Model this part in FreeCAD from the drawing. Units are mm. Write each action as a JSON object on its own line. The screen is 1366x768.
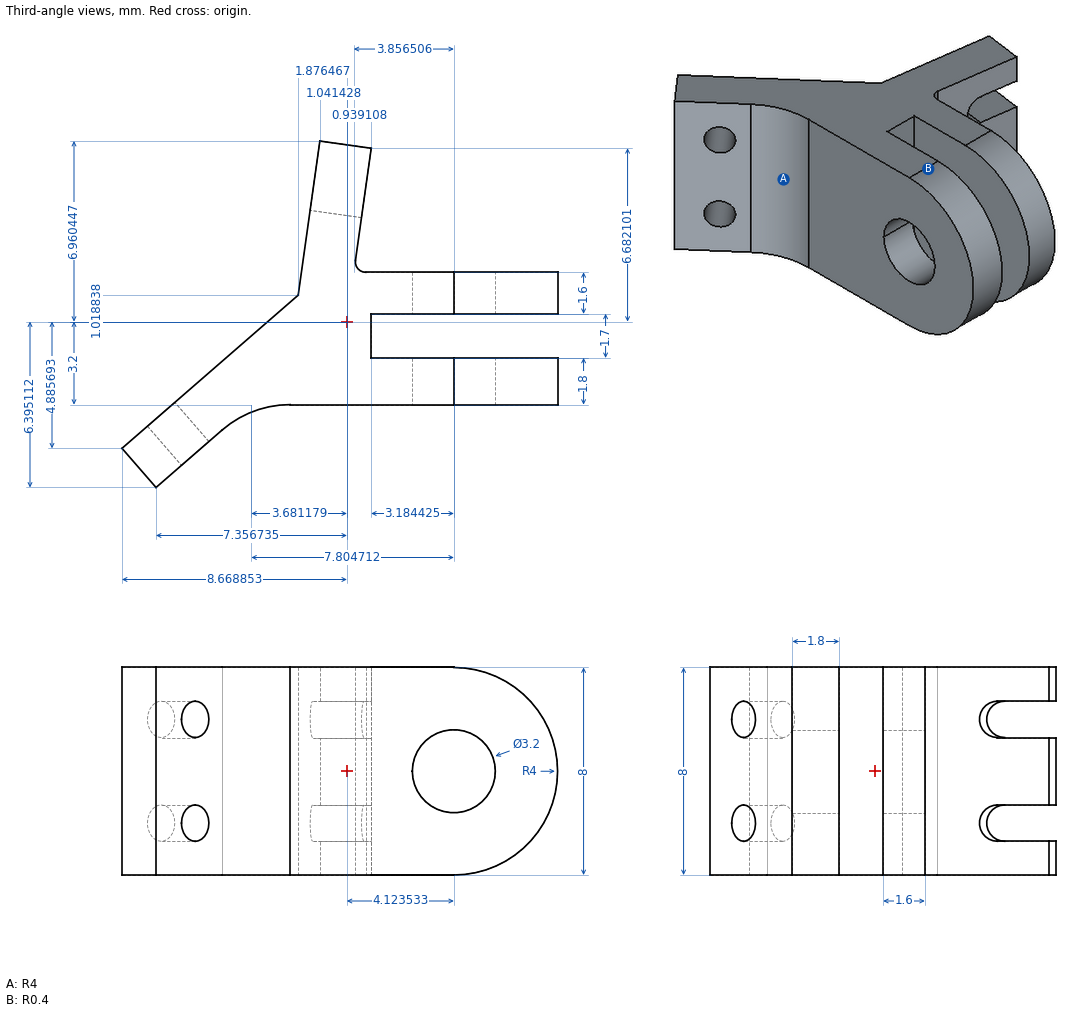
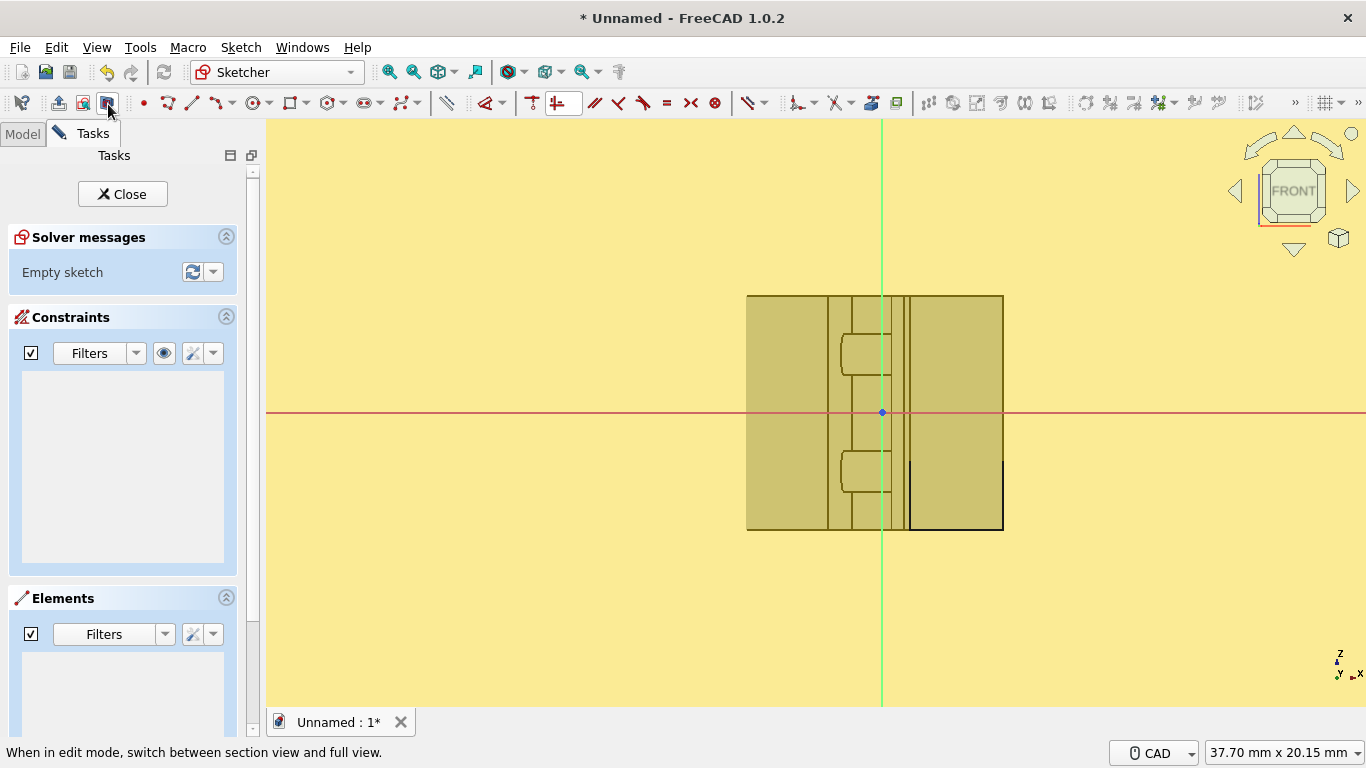
{"action": "scroll", "coordinate": [1201, 413], "scroll_direction": "up", "scroll_amount": 2}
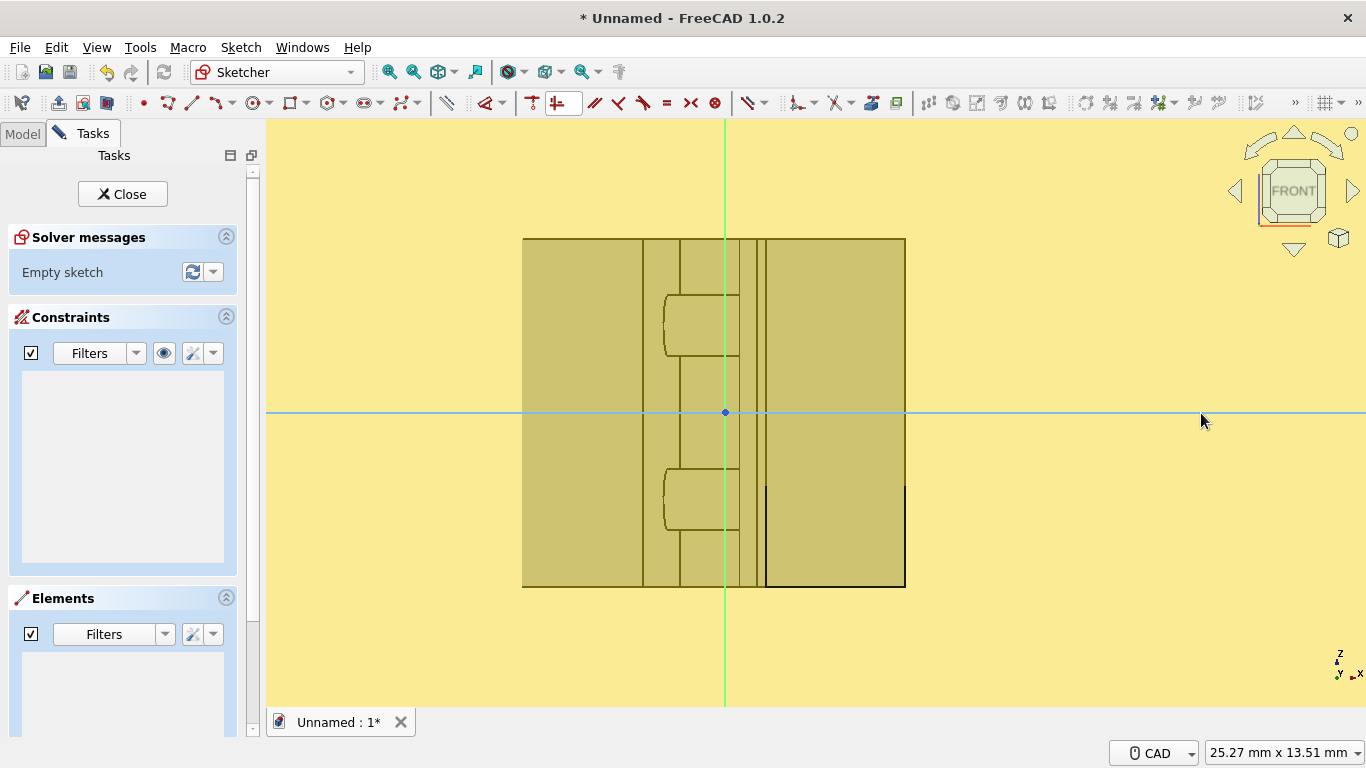
{"action": "left_click", "coordinate": [192, 104]}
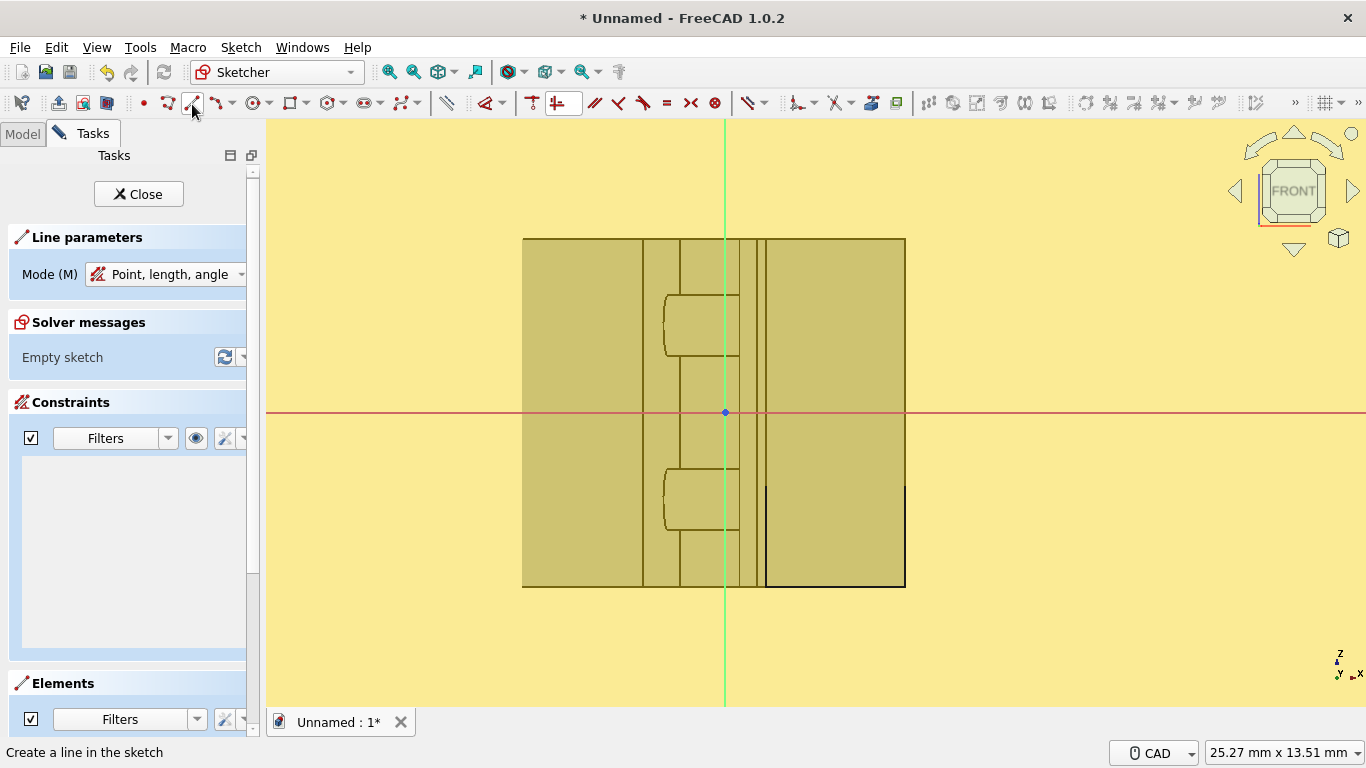
{"action": "left_click", "coordinate": [905, 587]}
{"action": "left_click", "coordinate": [905, 239]}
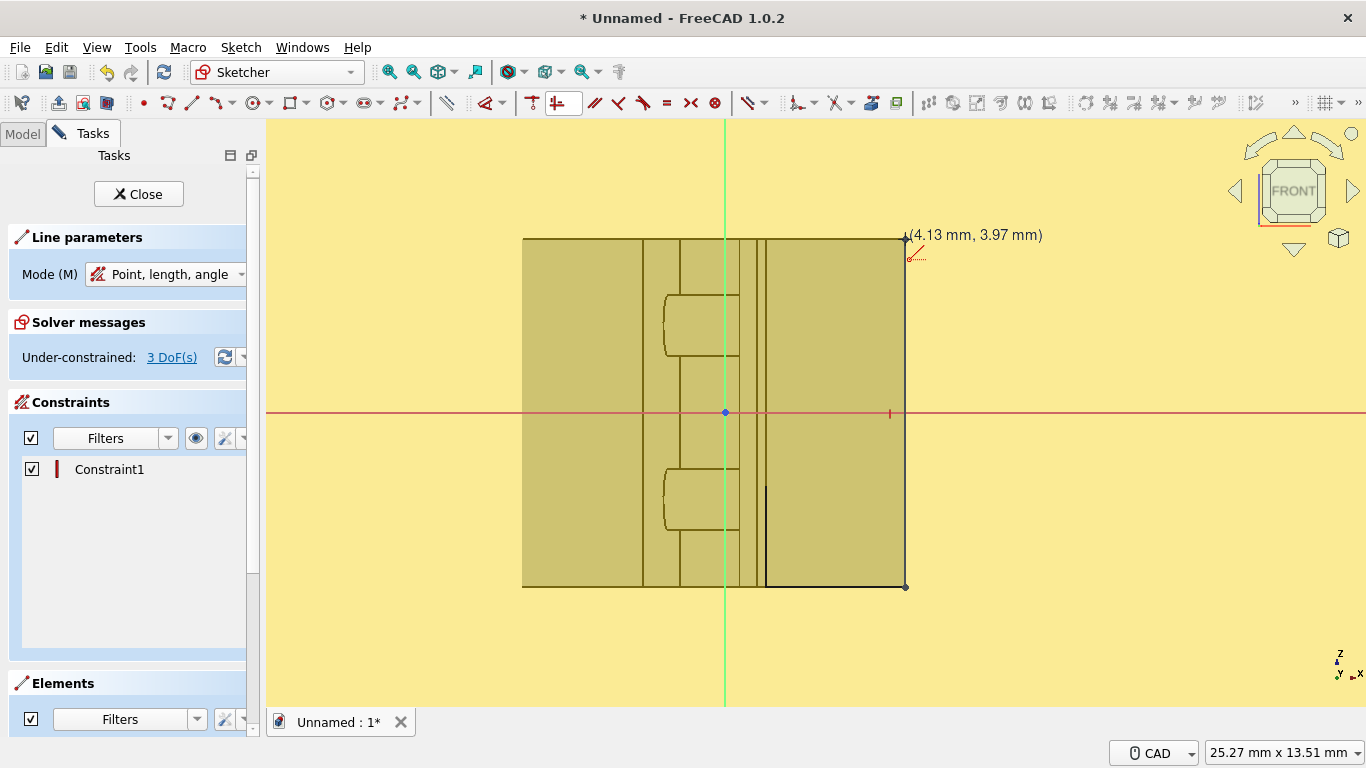
{"action": "left_click", "coordinate": [216, 104]}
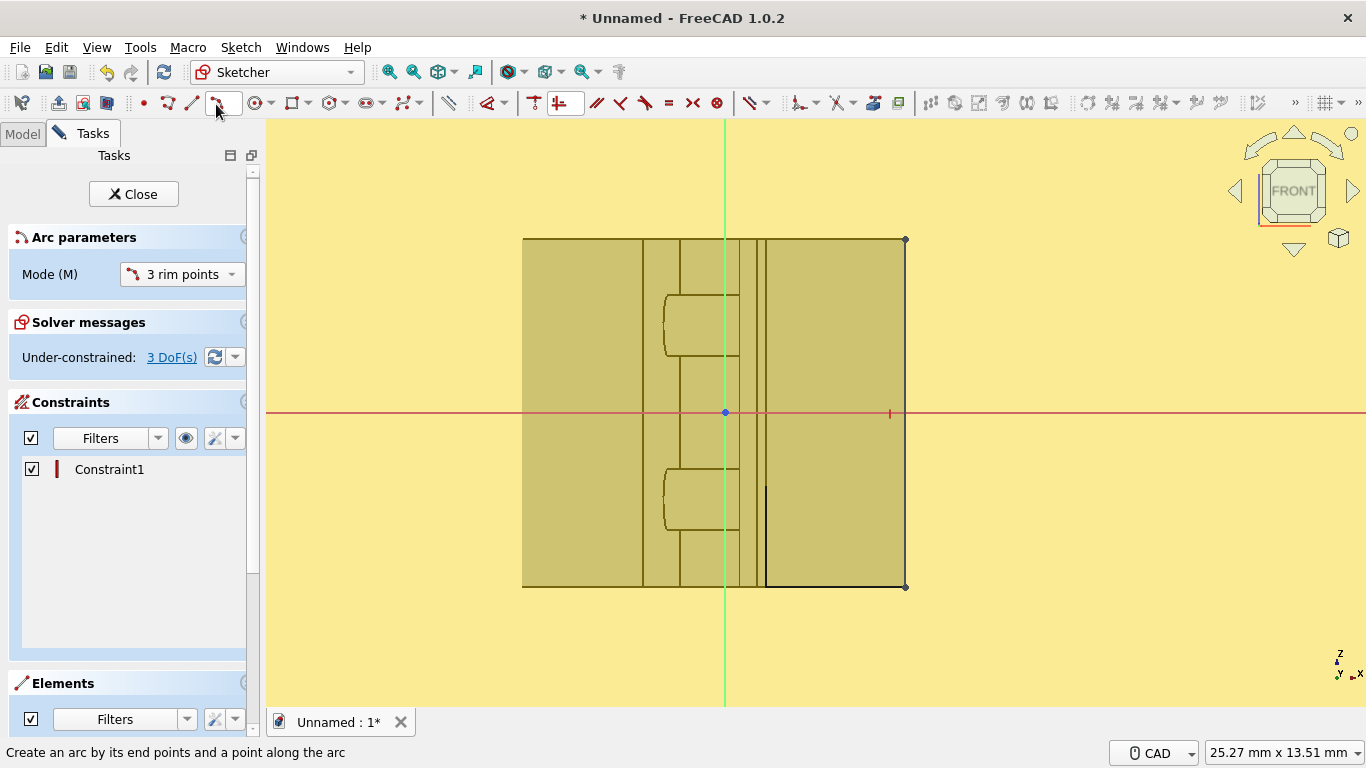
{"action": "left_click", "coordinate": [905, 240]}
{"action": "left_click", "coordinate": [905, 588]}
{"action": "left_click", "coordinate": [1070, 467]}
{"action": "key", "text": "Escape"}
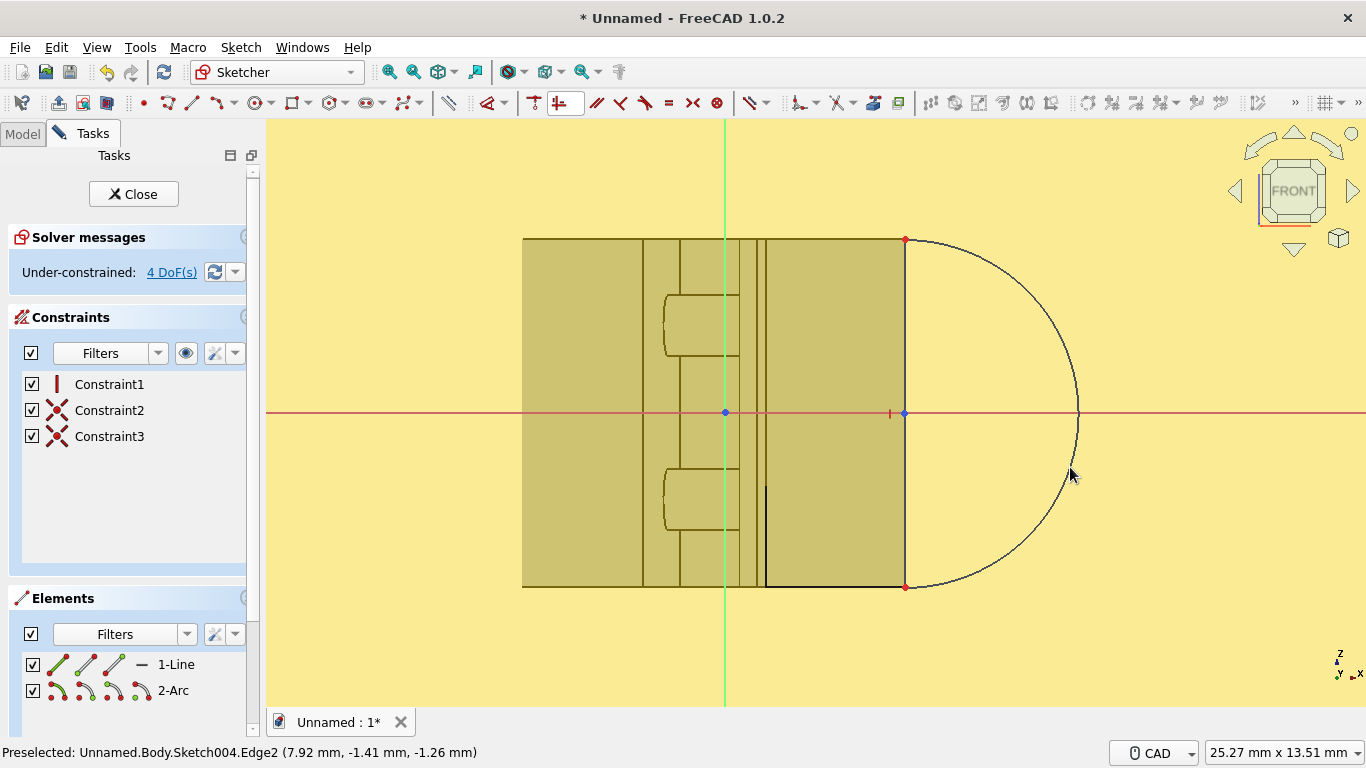
{"action": "left_click", "coordinate": [905, 414]}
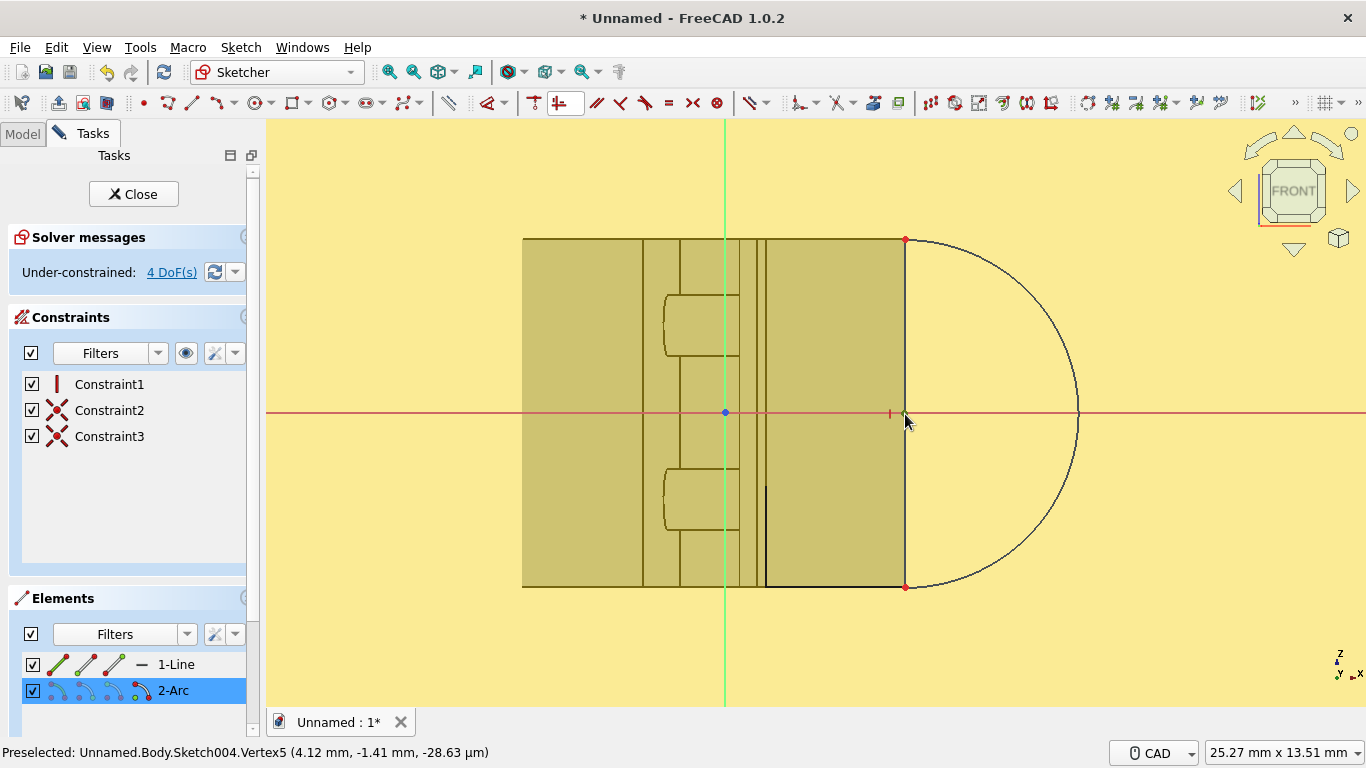
{"action": "left_click", "coordinate": [359, 413]}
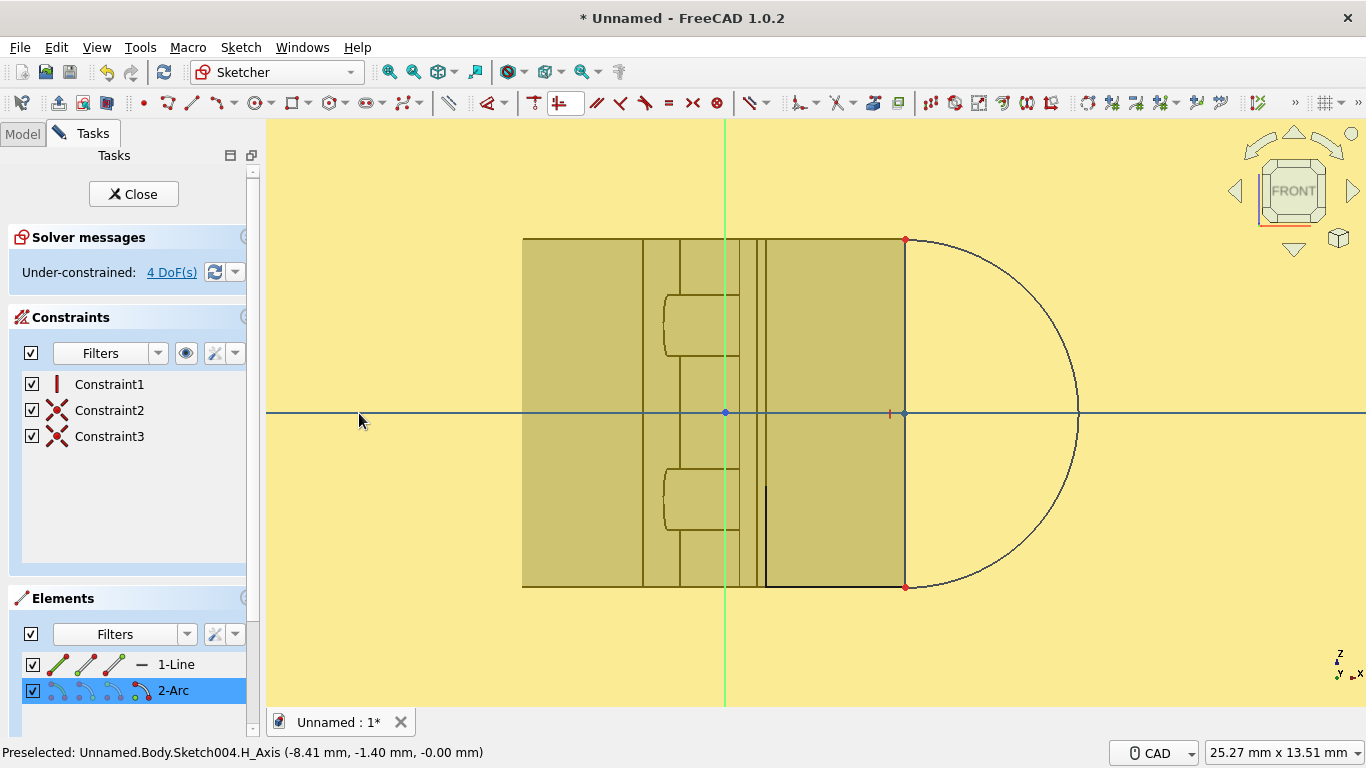
{"action": "left_click", "coordinate": [534, 104]}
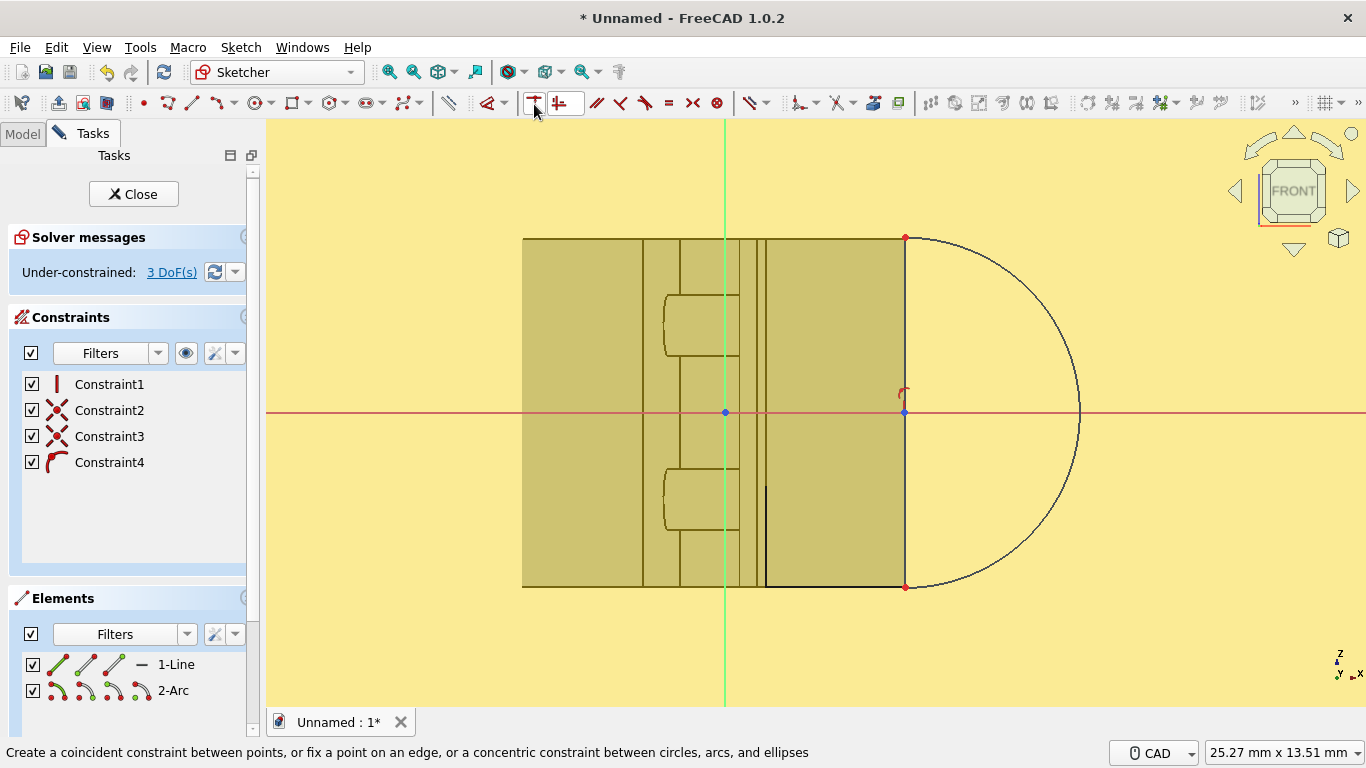
{"action": "left_click", "coordinate": [488, 104]}